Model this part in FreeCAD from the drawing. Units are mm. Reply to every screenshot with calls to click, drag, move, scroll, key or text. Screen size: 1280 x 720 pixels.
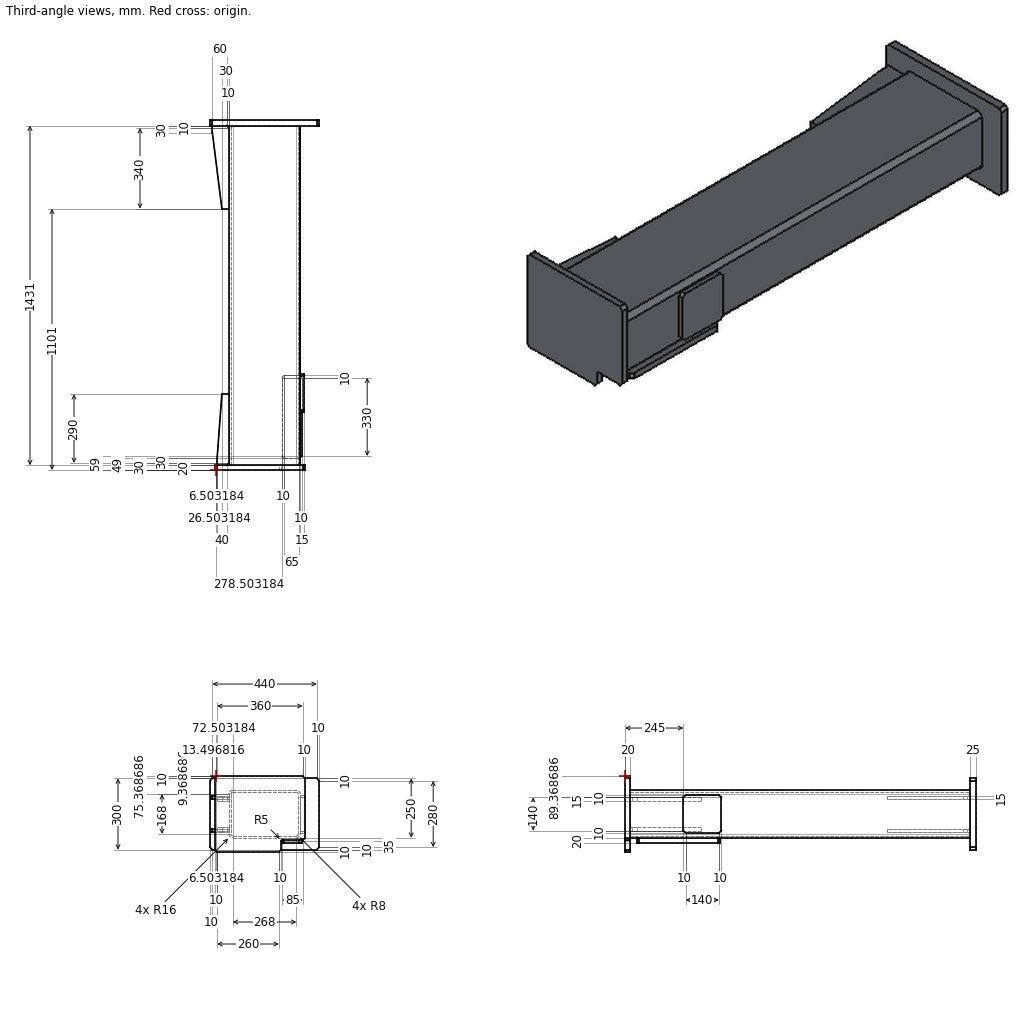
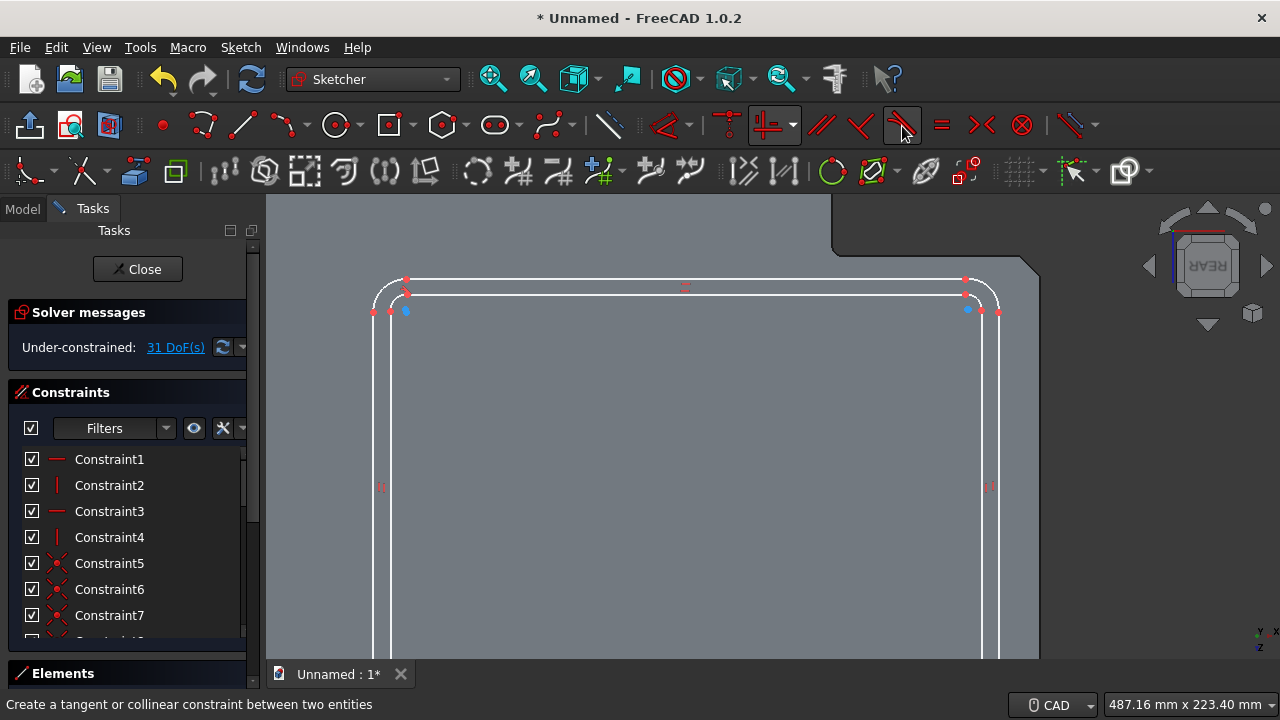
click(798, 279)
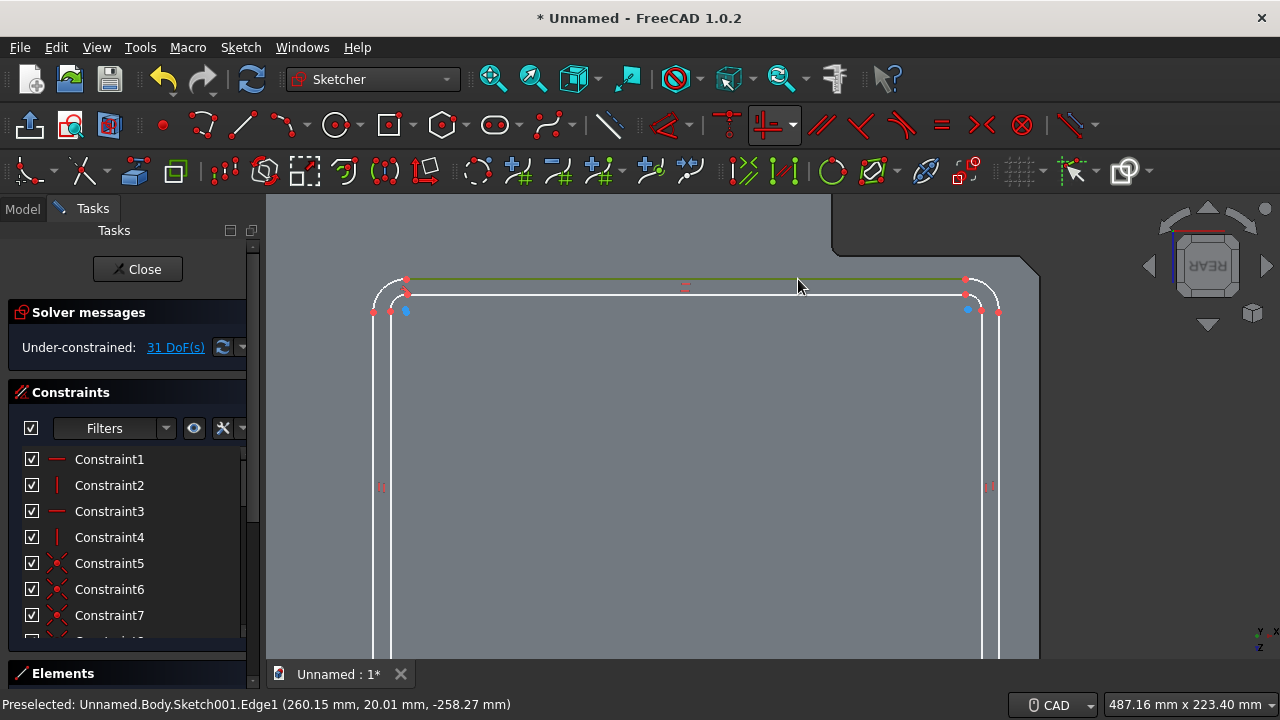
click(996, 297)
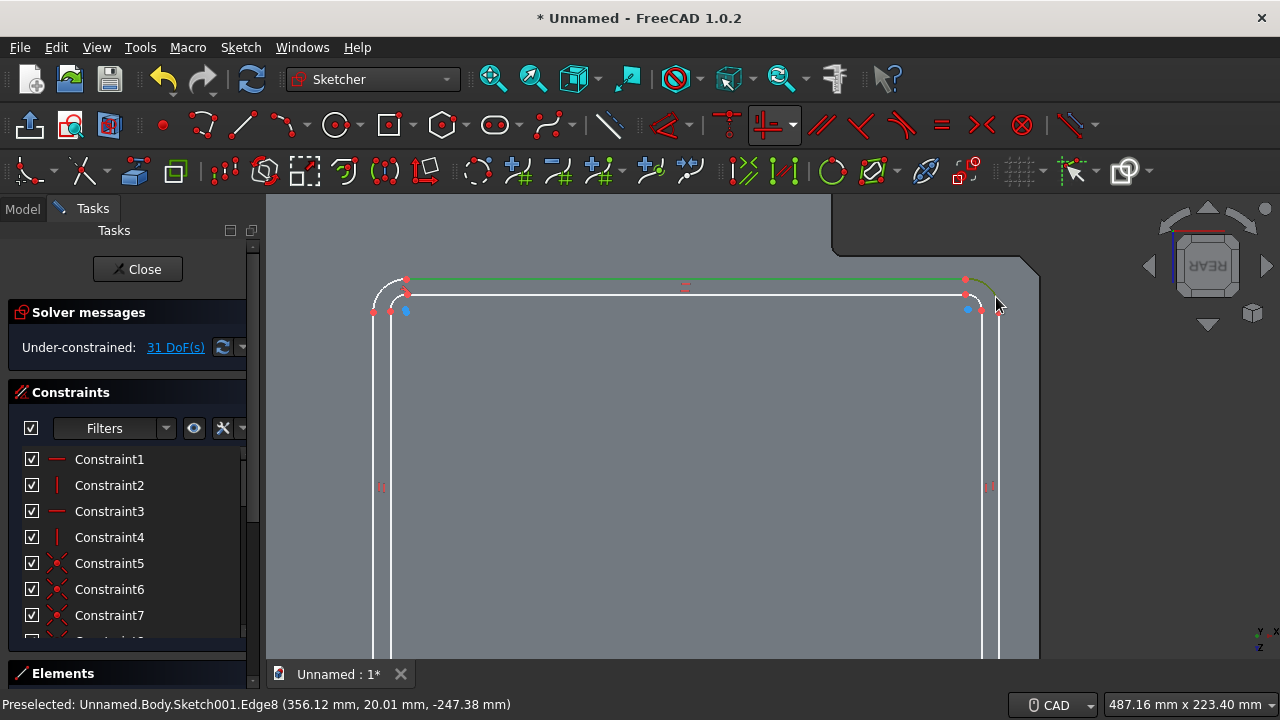
key(t)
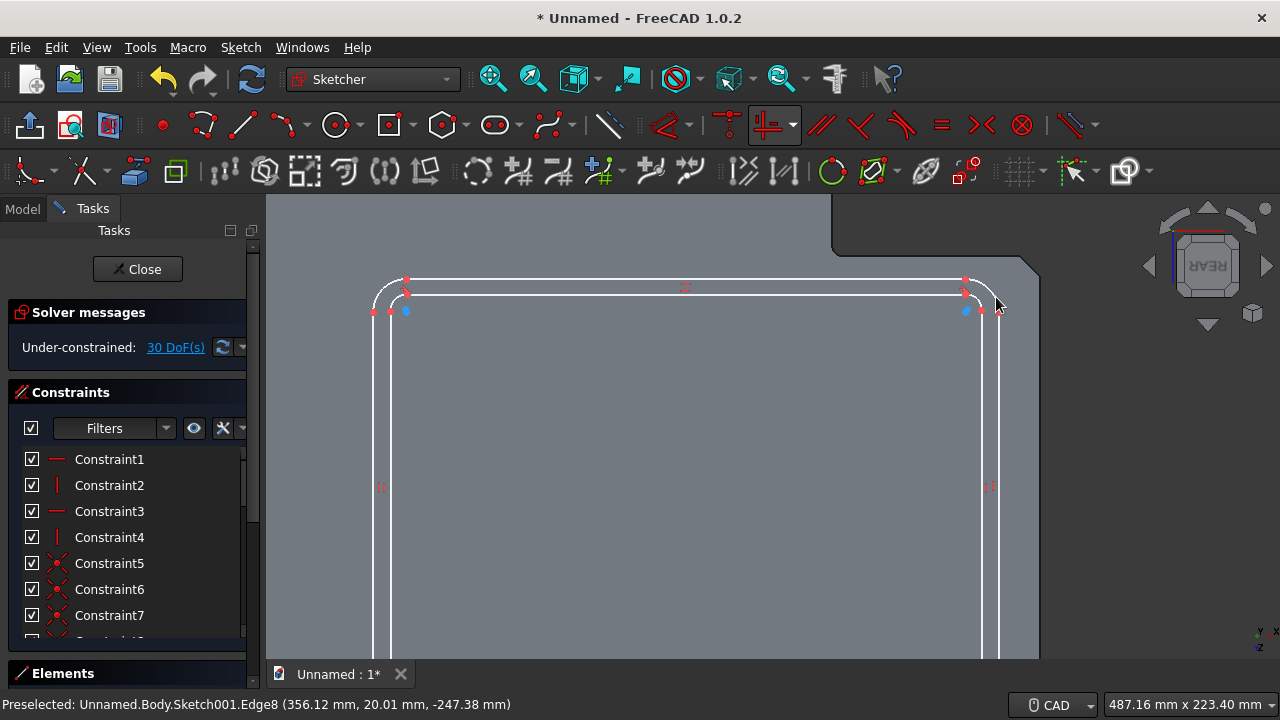
click(373, 417)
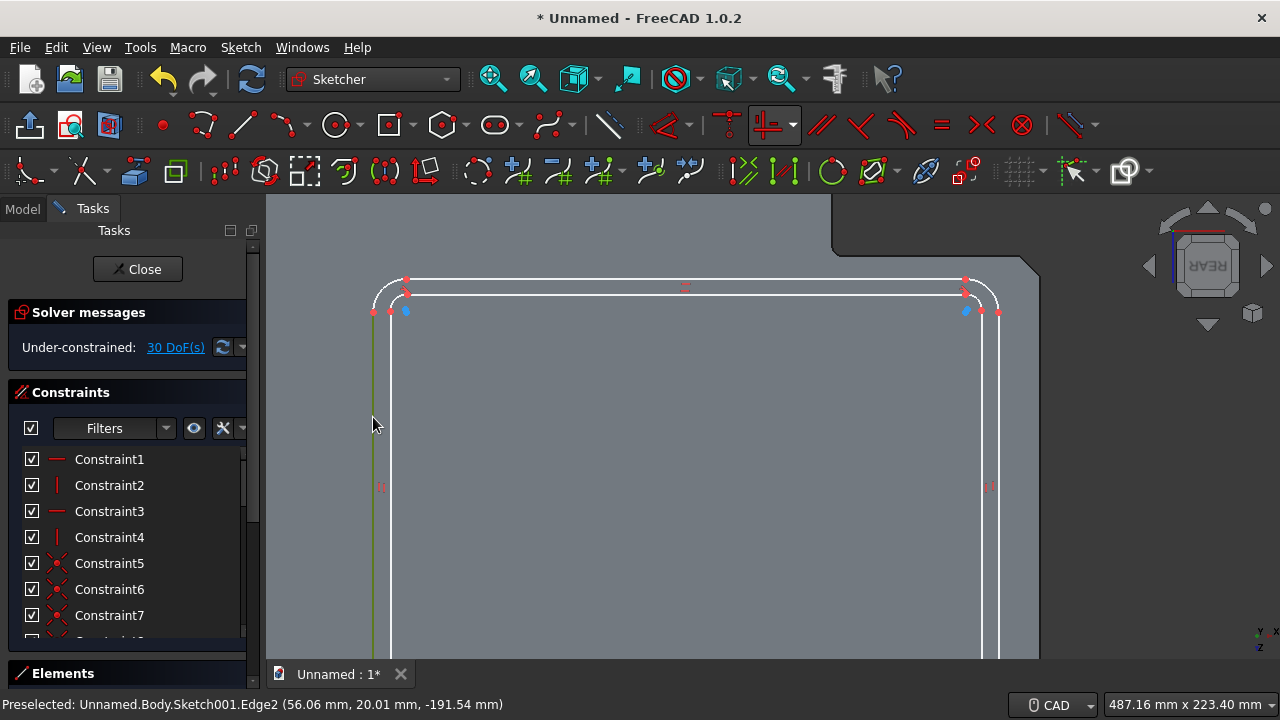
click(391, 283)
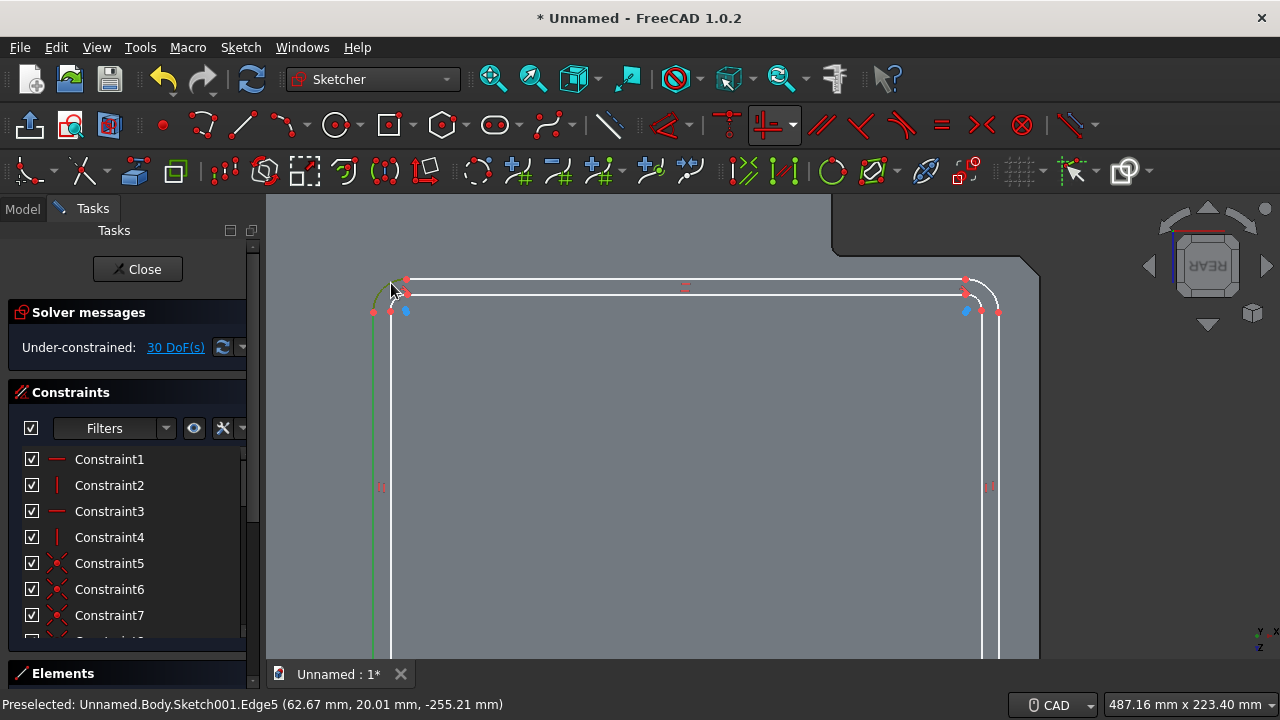
click(902, 126)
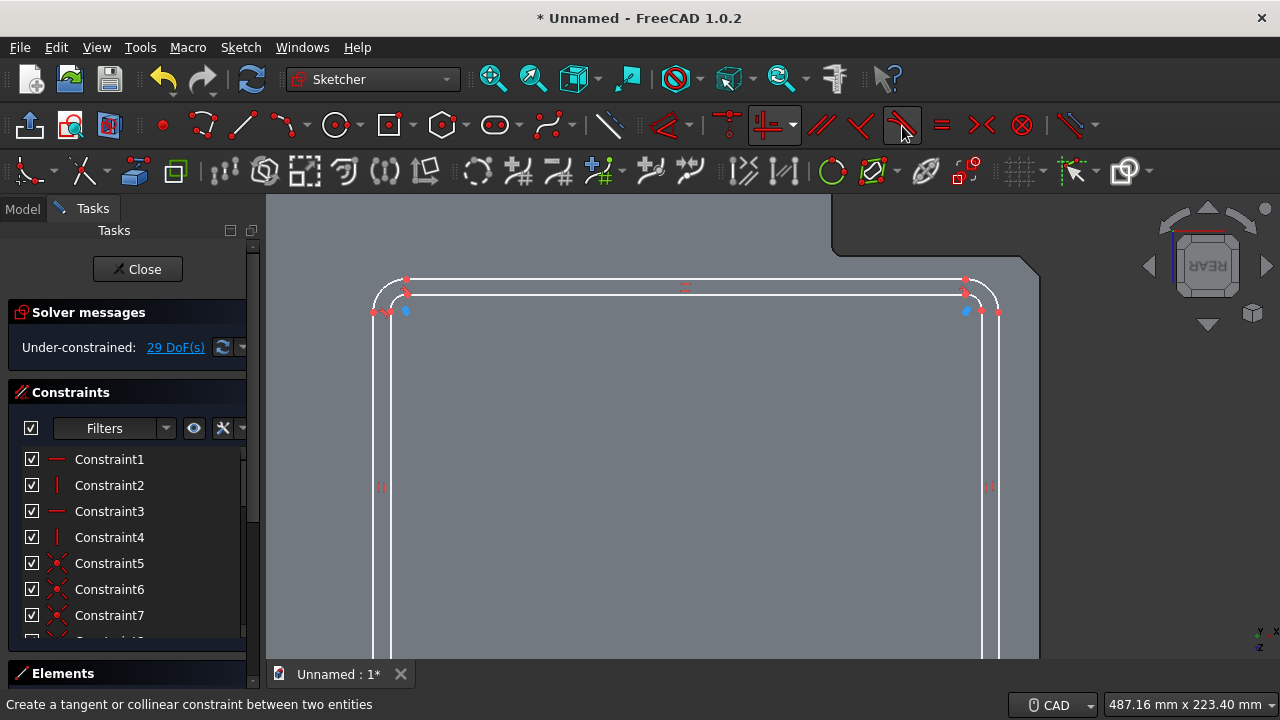
click(373, 417)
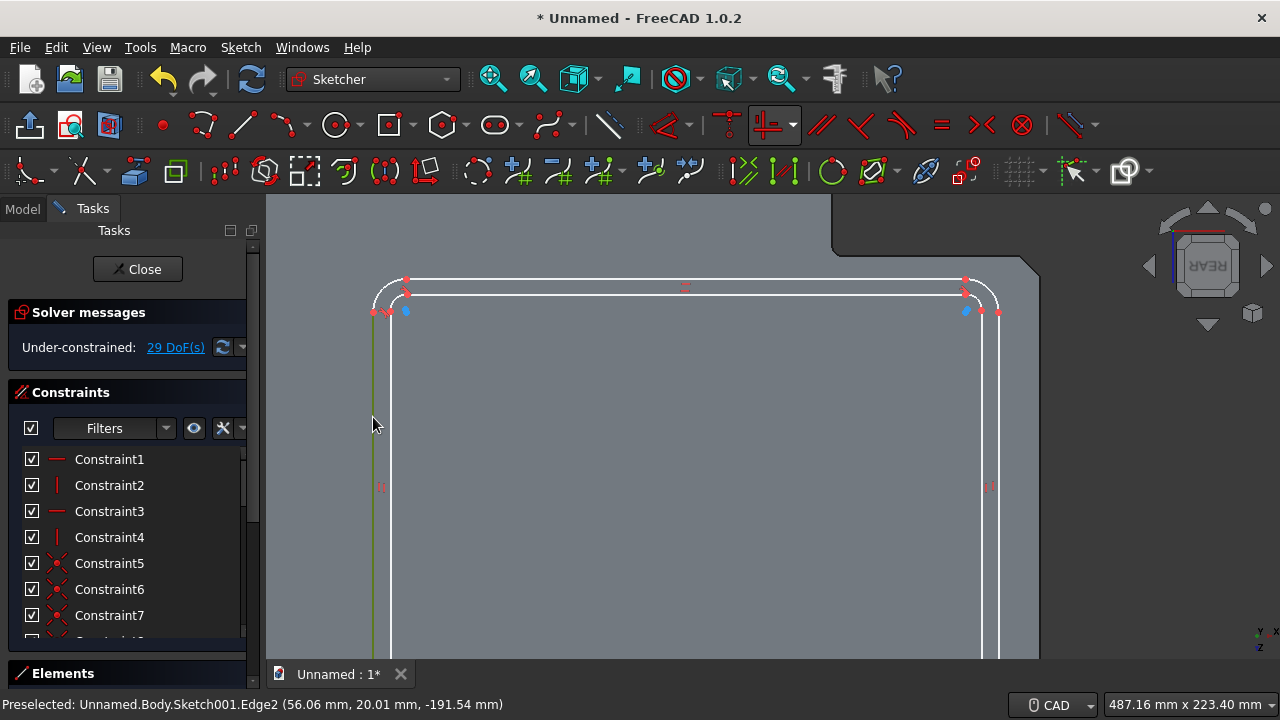
scroll(798, 280, down, 3)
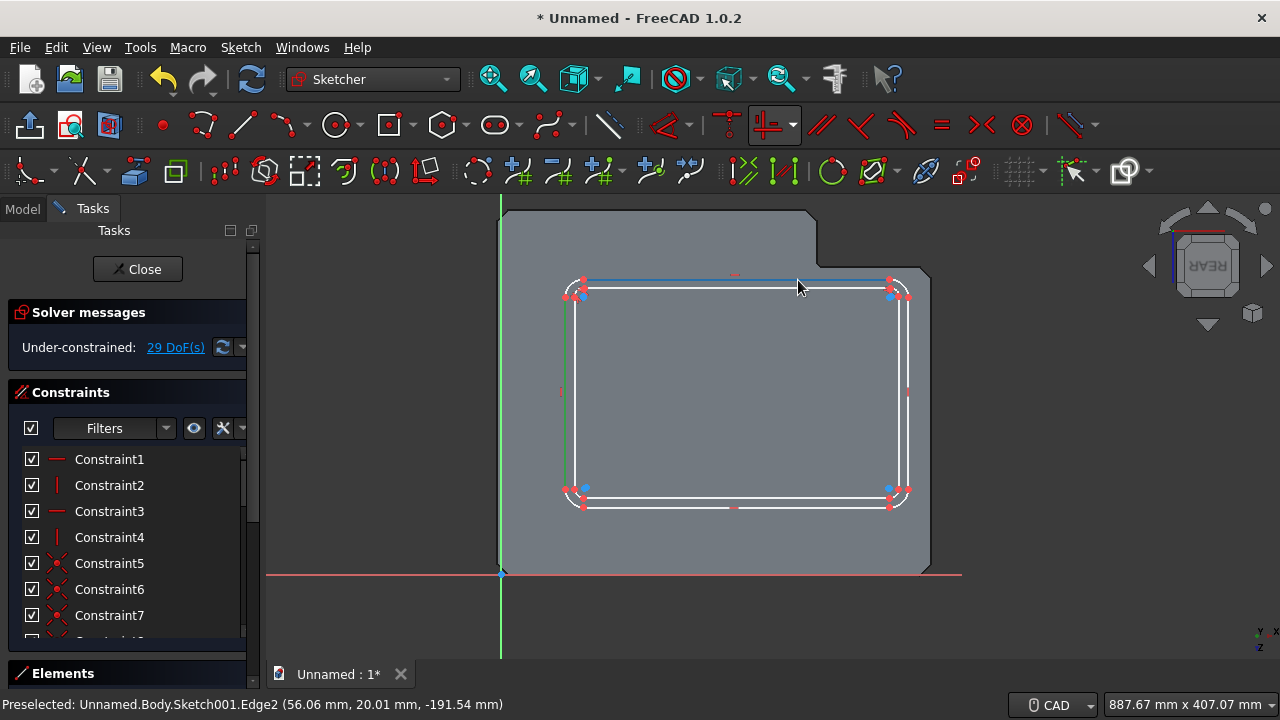
scroll(568, 498, up, 3)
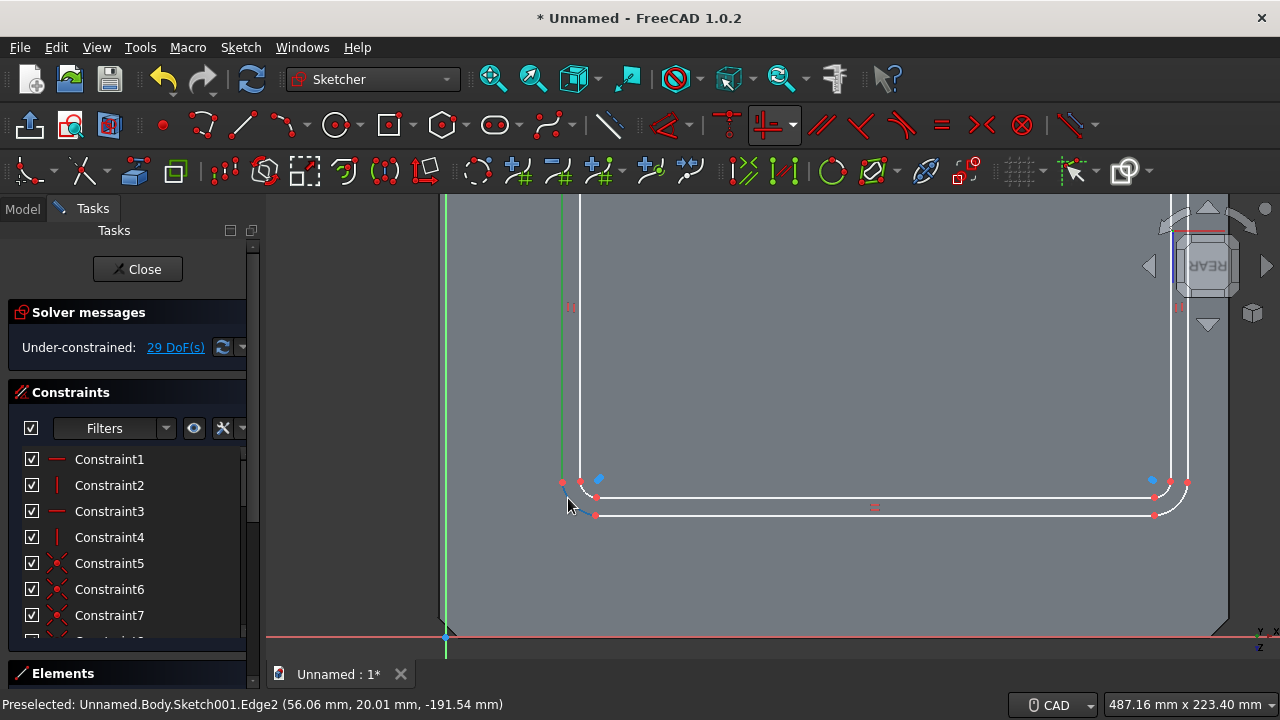
click(567, 497)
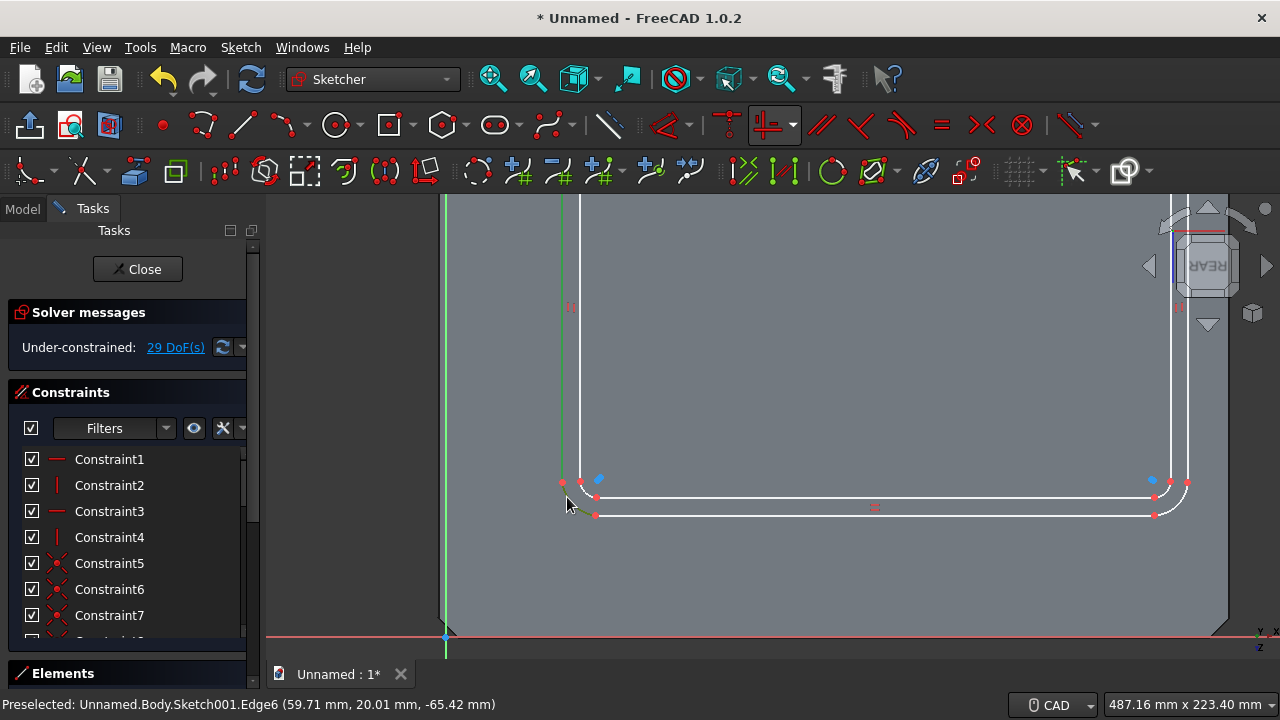
click(902, 126)